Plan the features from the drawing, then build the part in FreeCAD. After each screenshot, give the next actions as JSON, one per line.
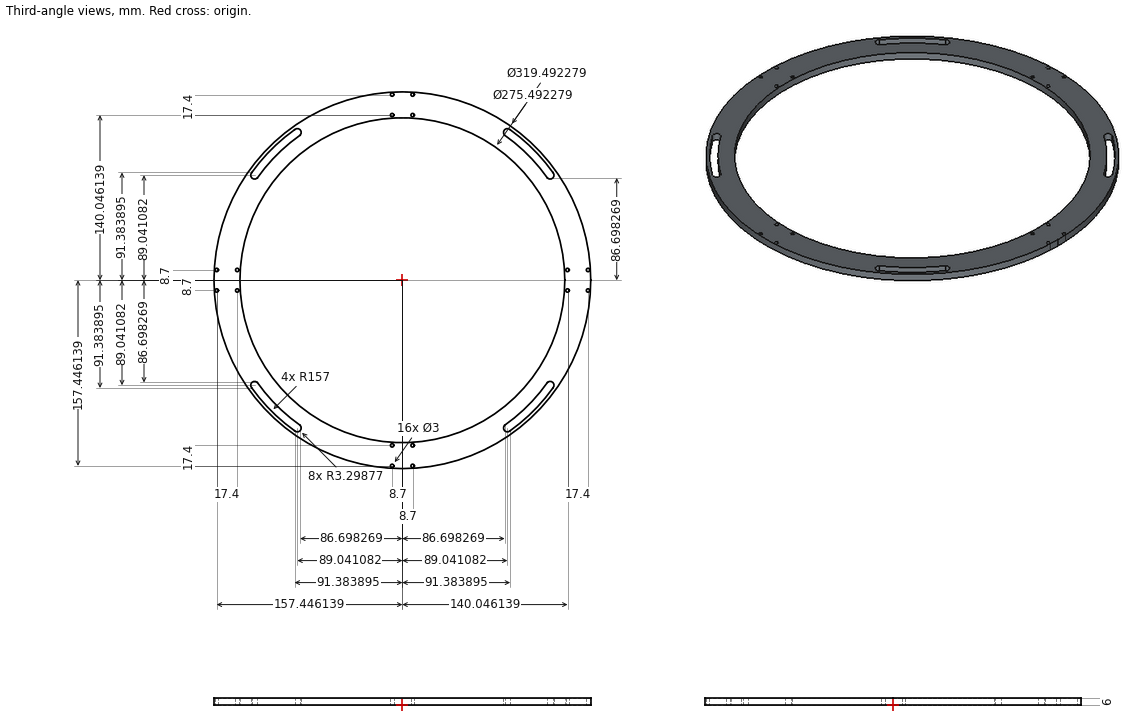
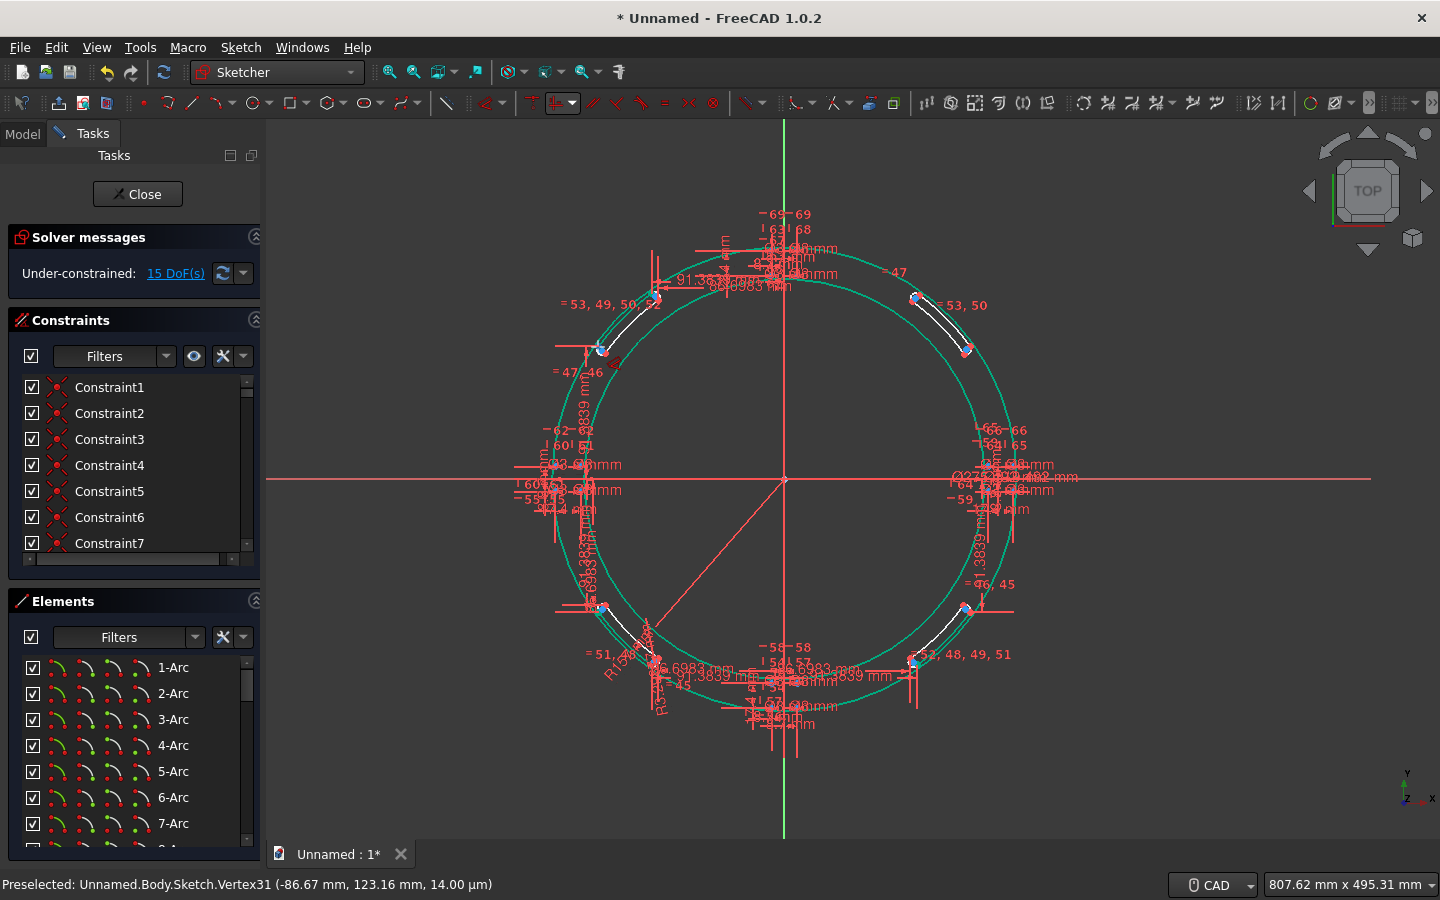
{"action": "scroll", "coordinate": [919, 295], "scroll_direction": "up", "scroll_amount": 5}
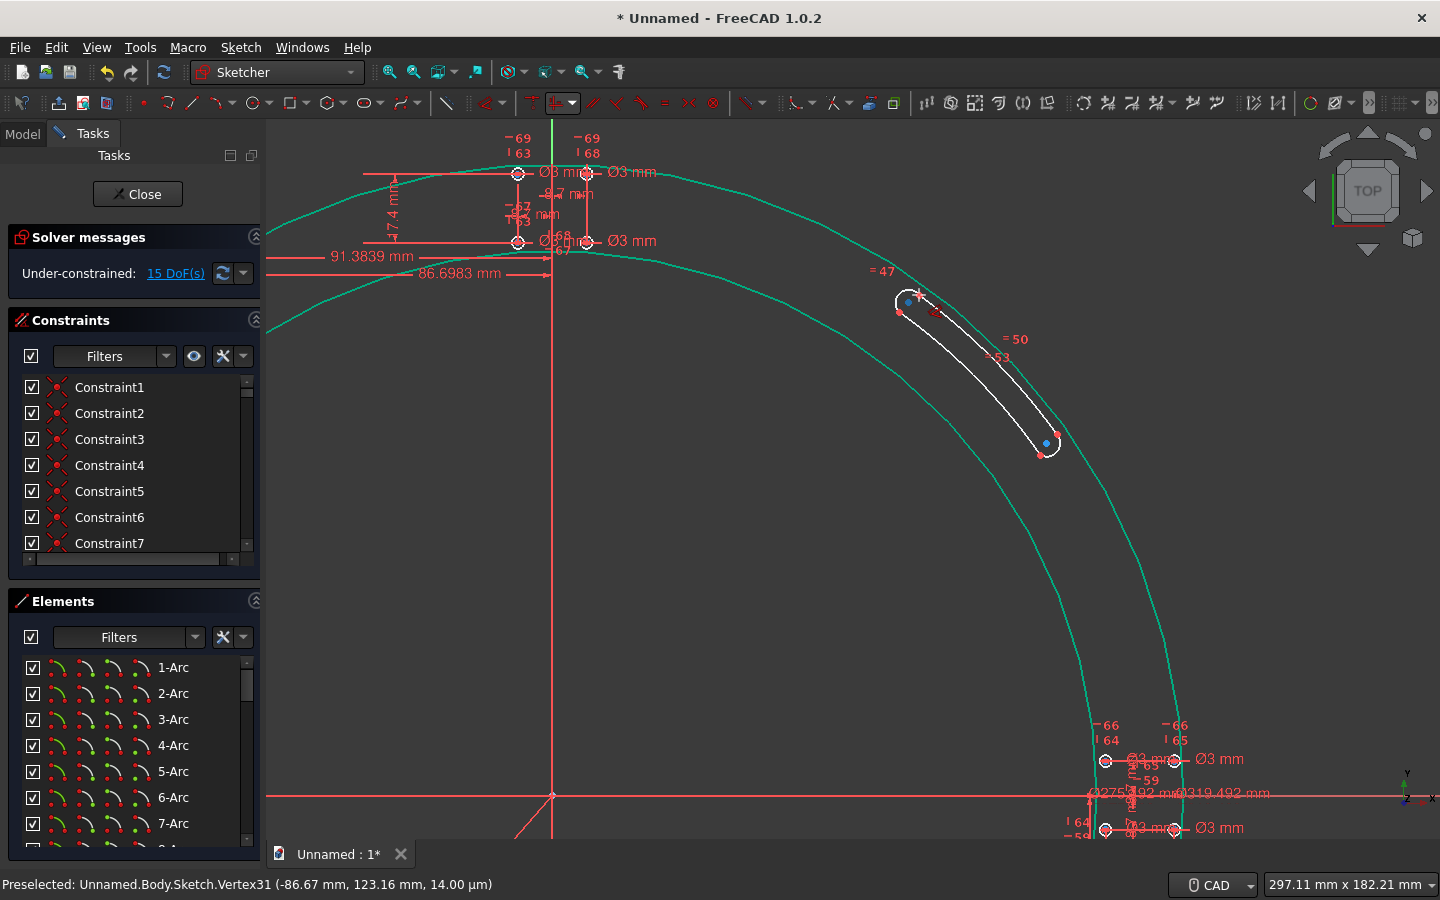
{"action": "left_click", "coordinate": [919, 295]}
{"action": "left_click", "coordinate": [736, 261]}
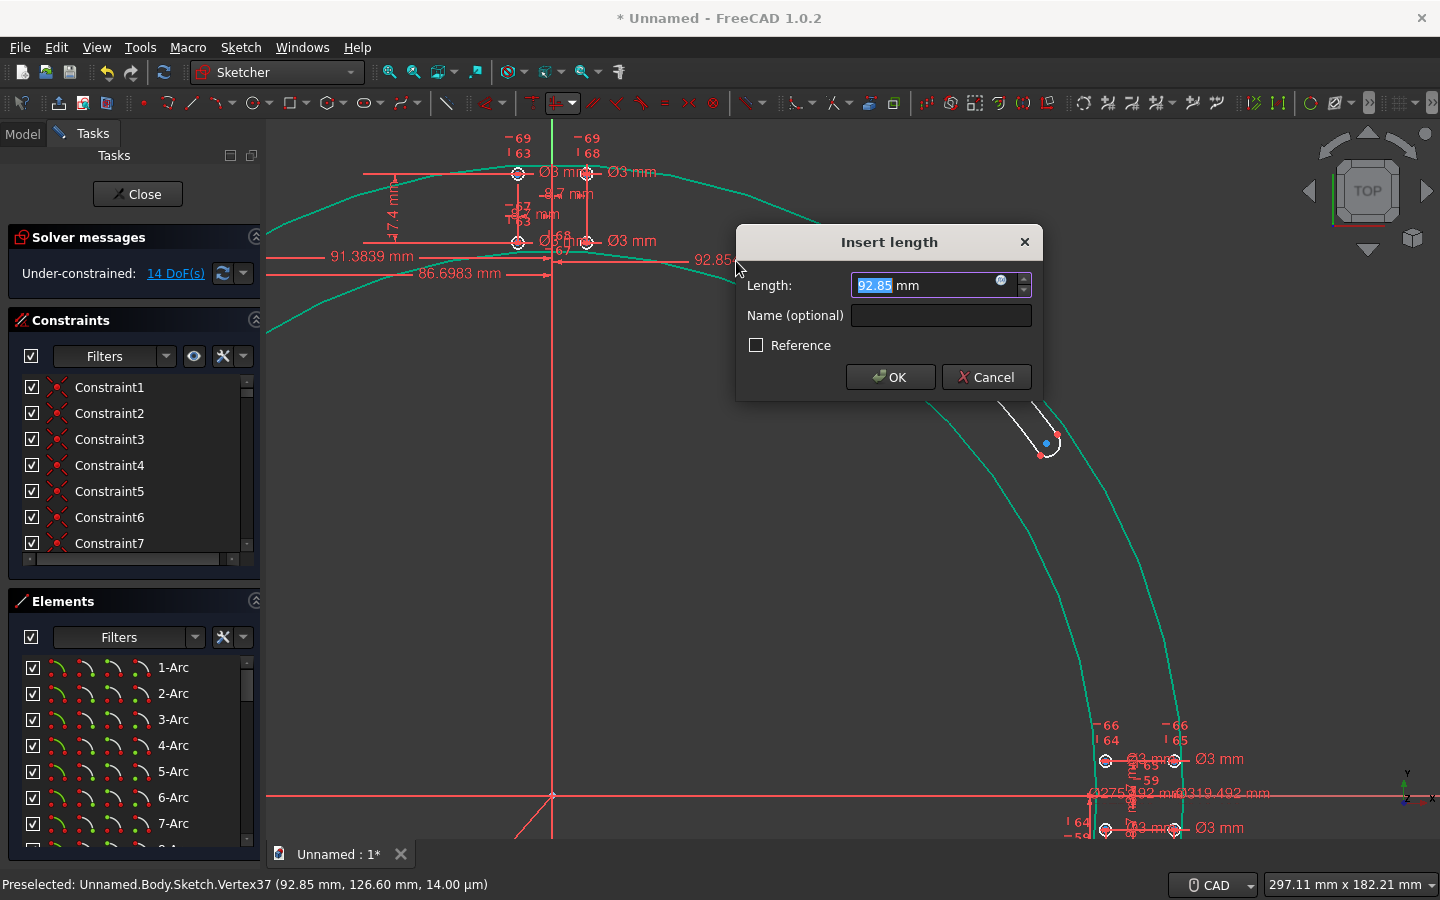
{"action": "type", "text": "91.383895"}
{"action": "key", "text": "Return"}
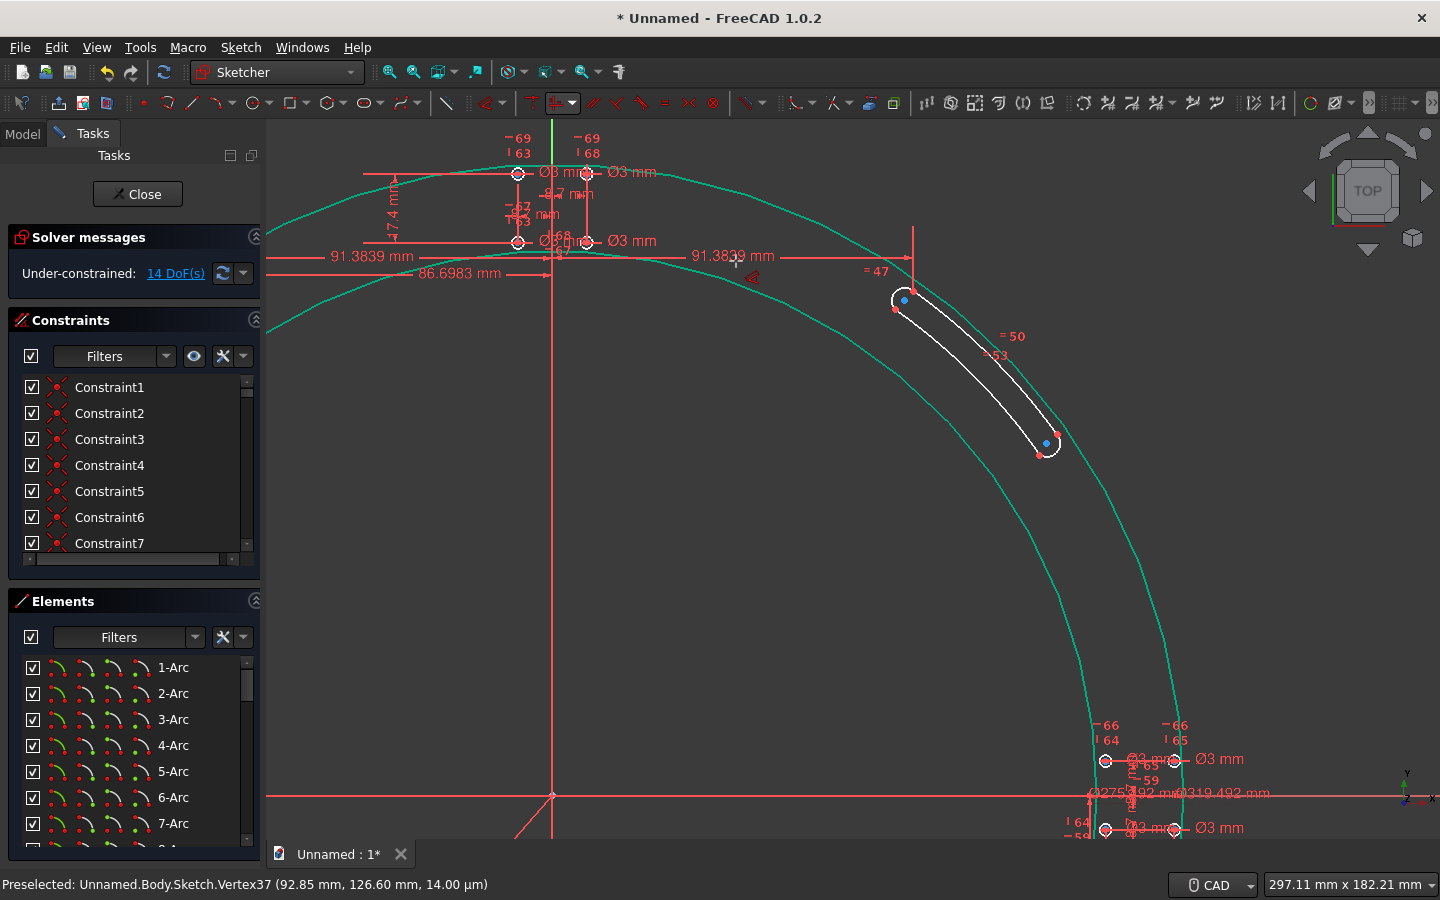
{"action": "left_click", "coordinate": [1057, 435]}
{"action": "left_click", "coordinate": [1091, 615]}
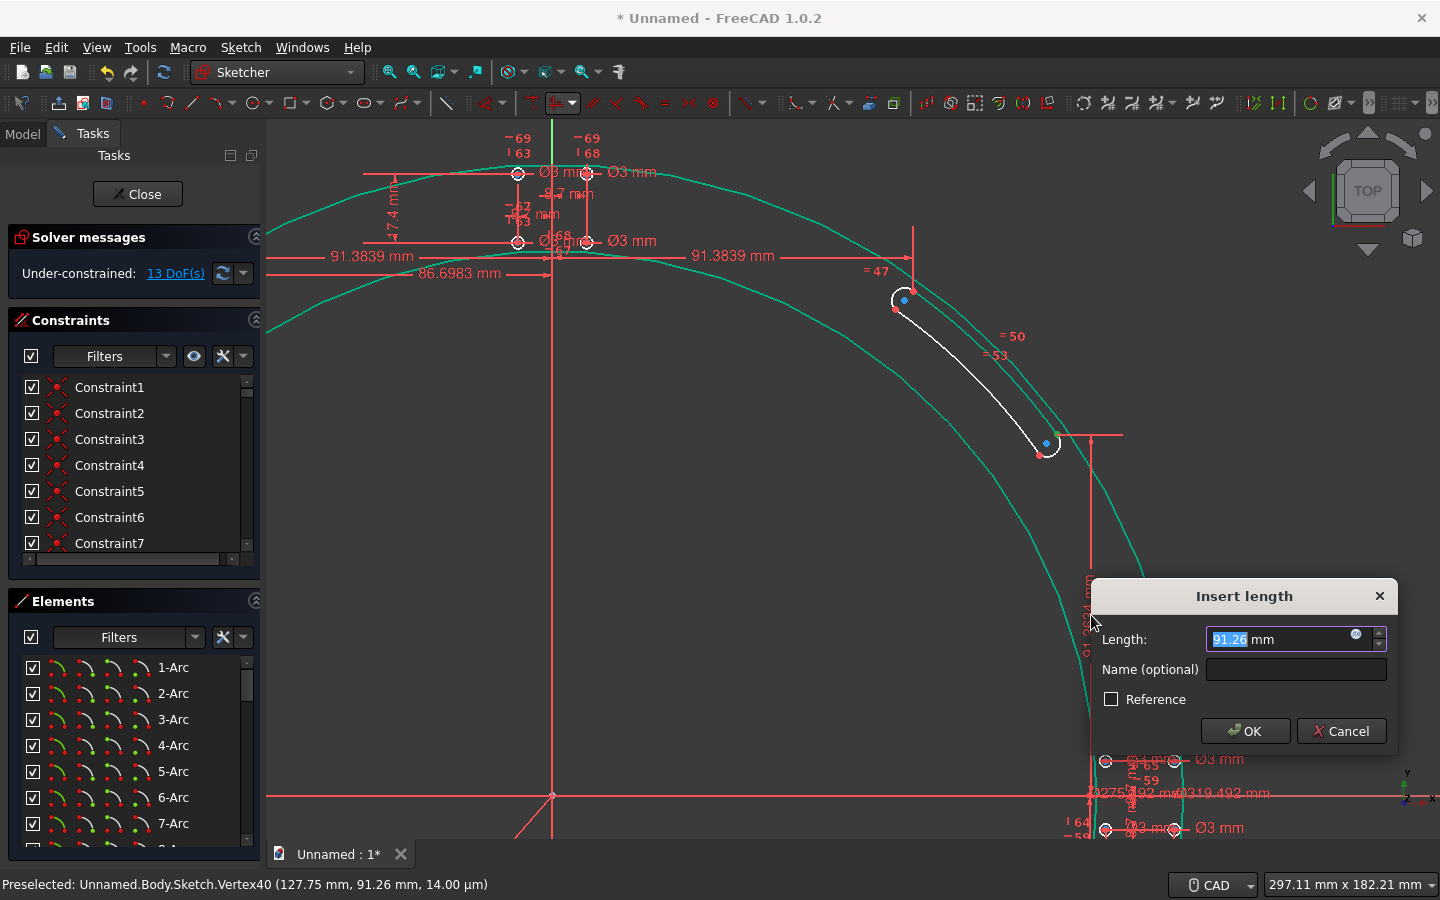
{"action": "type", "text": "91.383895"}
{"action": "key", "text": "Return"}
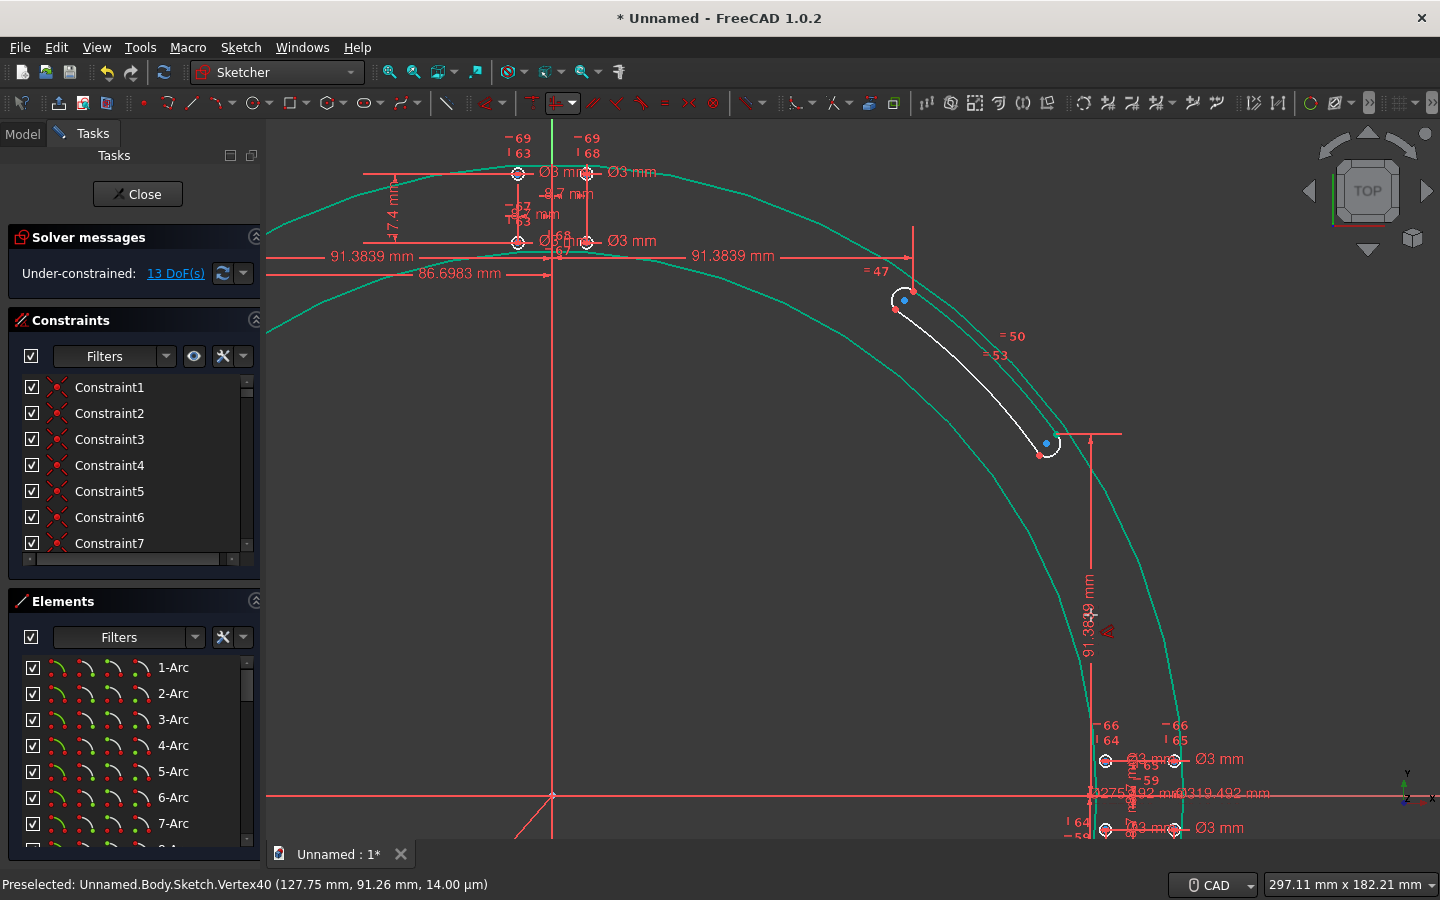
{"action": "left_click", "coordinate": [1040, 455]}
{"action": "left_click", "coordinate": [1074, 547]}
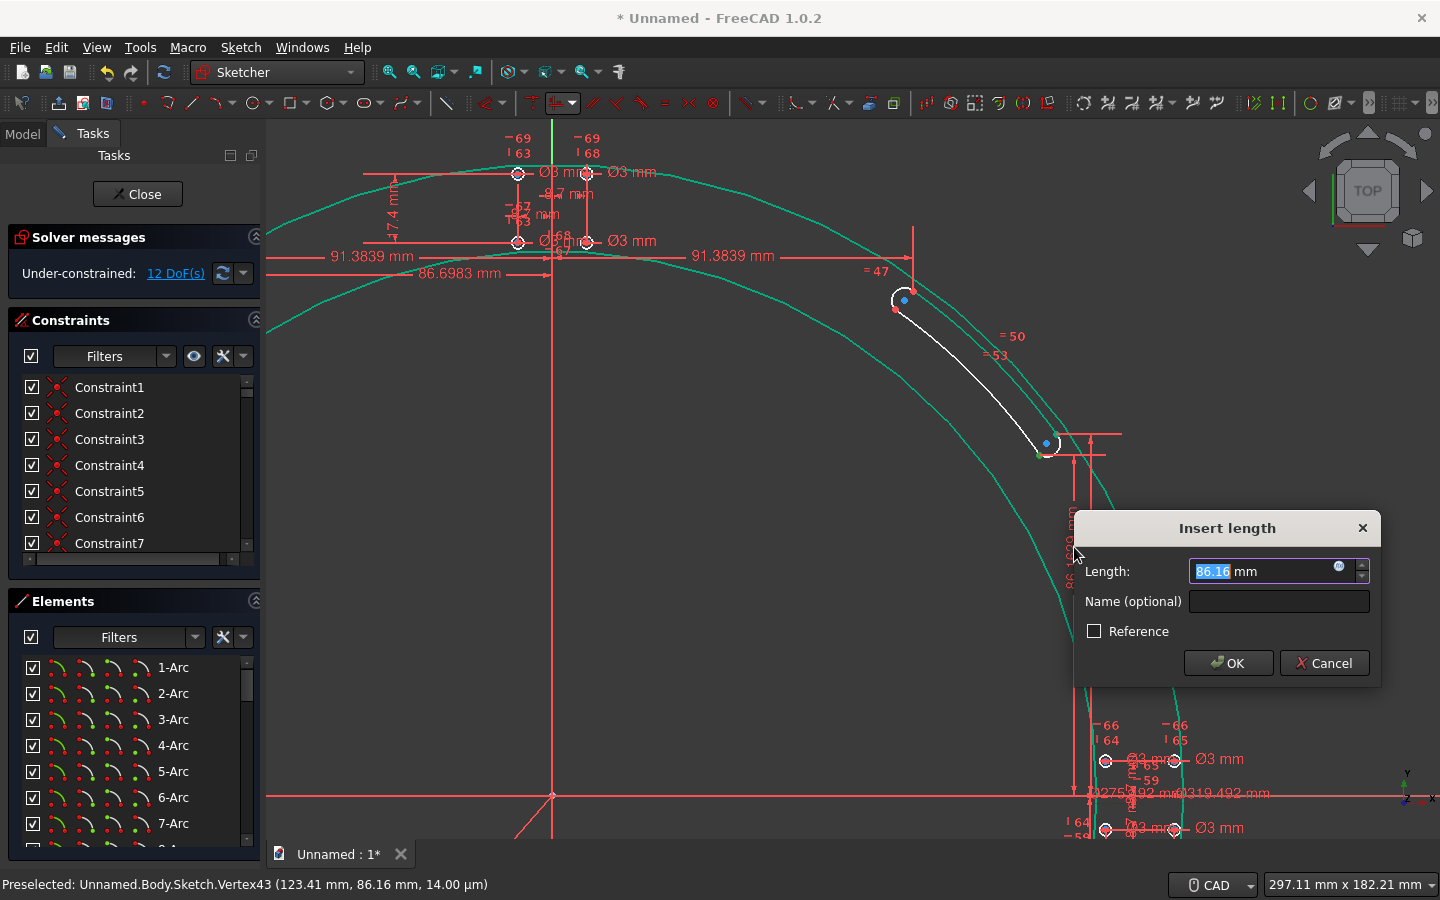
{"action": "type", "text": "86.698269"}
{"action": "key", "text": "Return"}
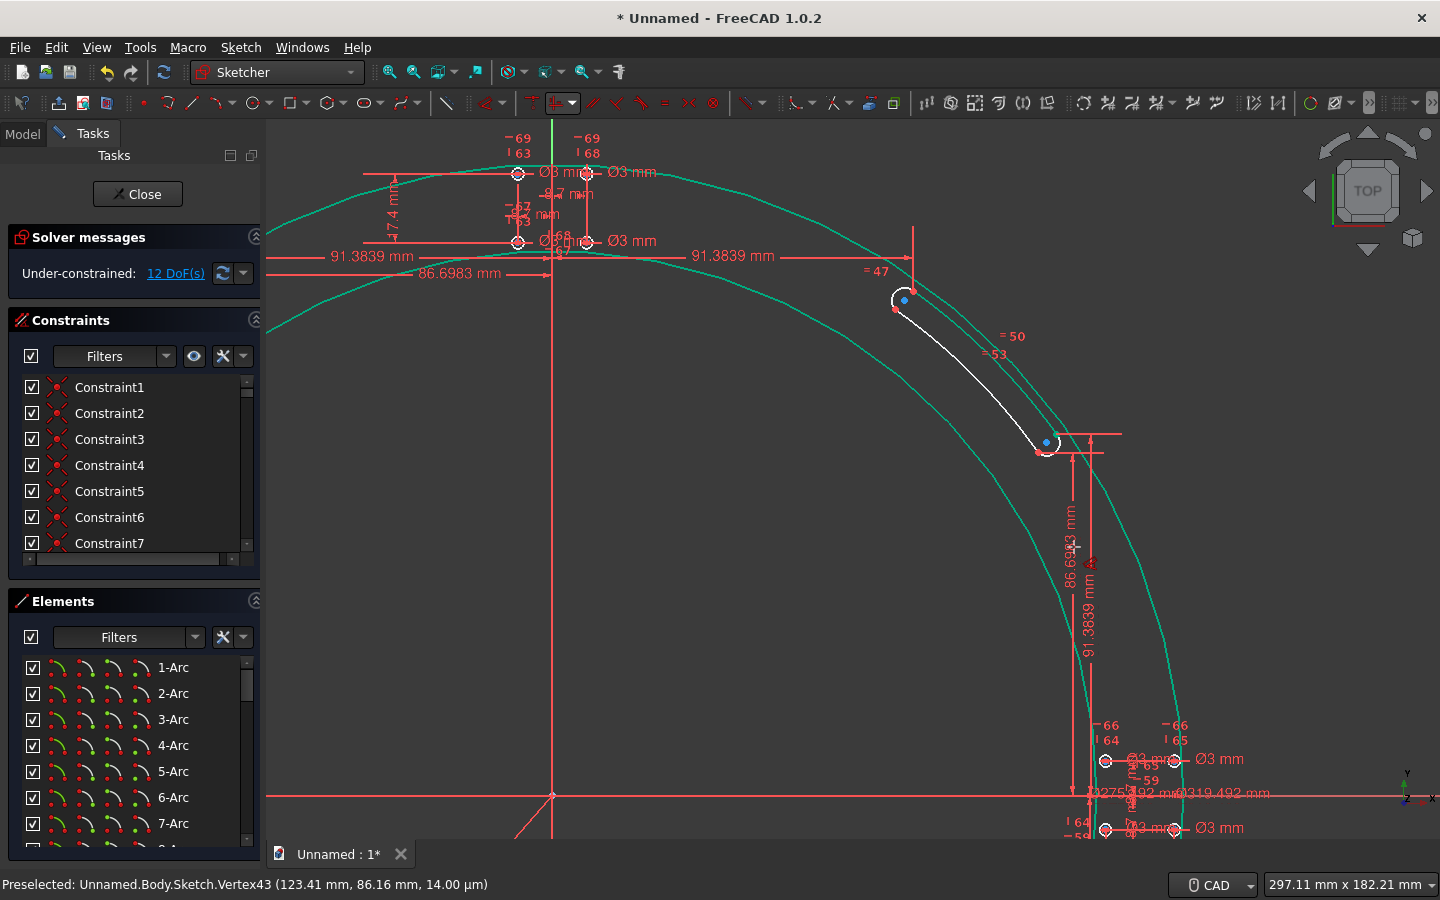
{"action": "scroll", "coordinate": [920, 295], "scroll_direction": "down", "scroll_amount": 5}